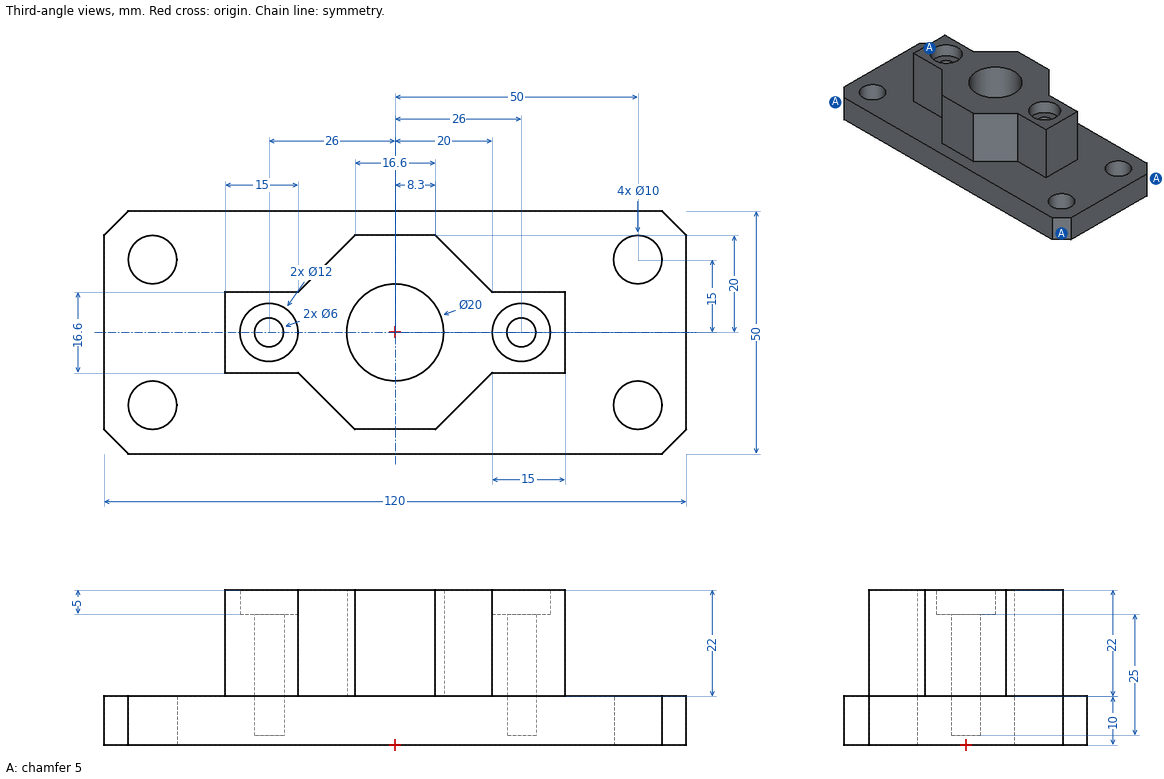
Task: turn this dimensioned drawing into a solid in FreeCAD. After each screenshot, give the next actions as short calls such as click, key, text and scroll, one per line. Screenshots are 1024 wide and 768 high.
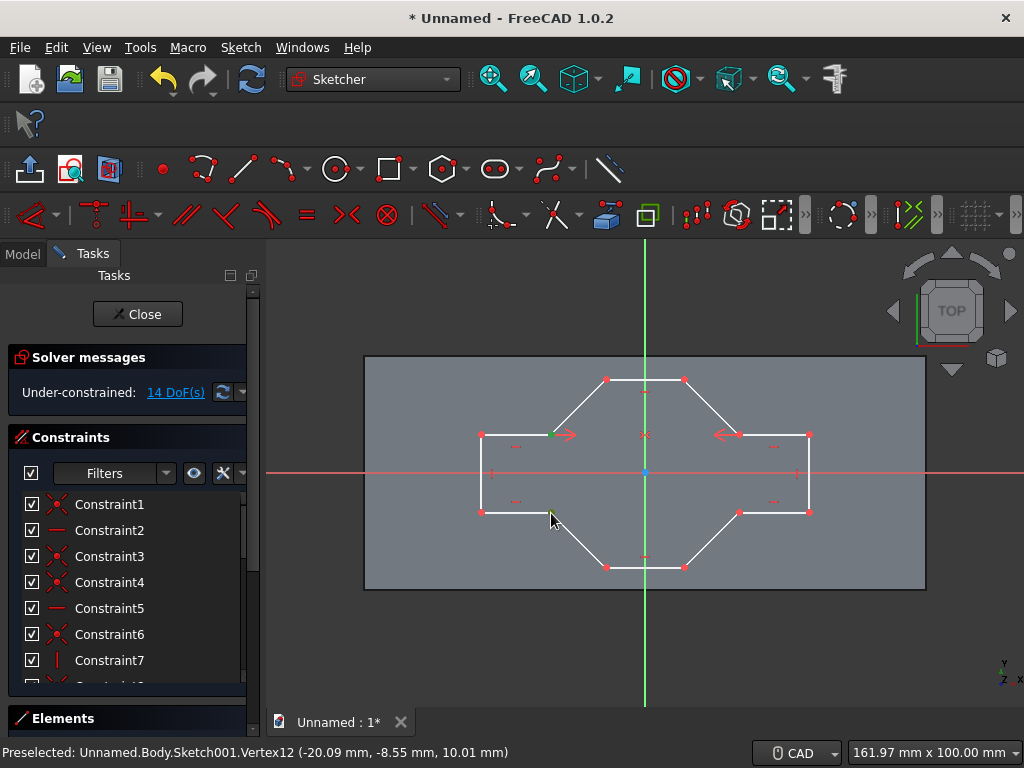
click(334, 473)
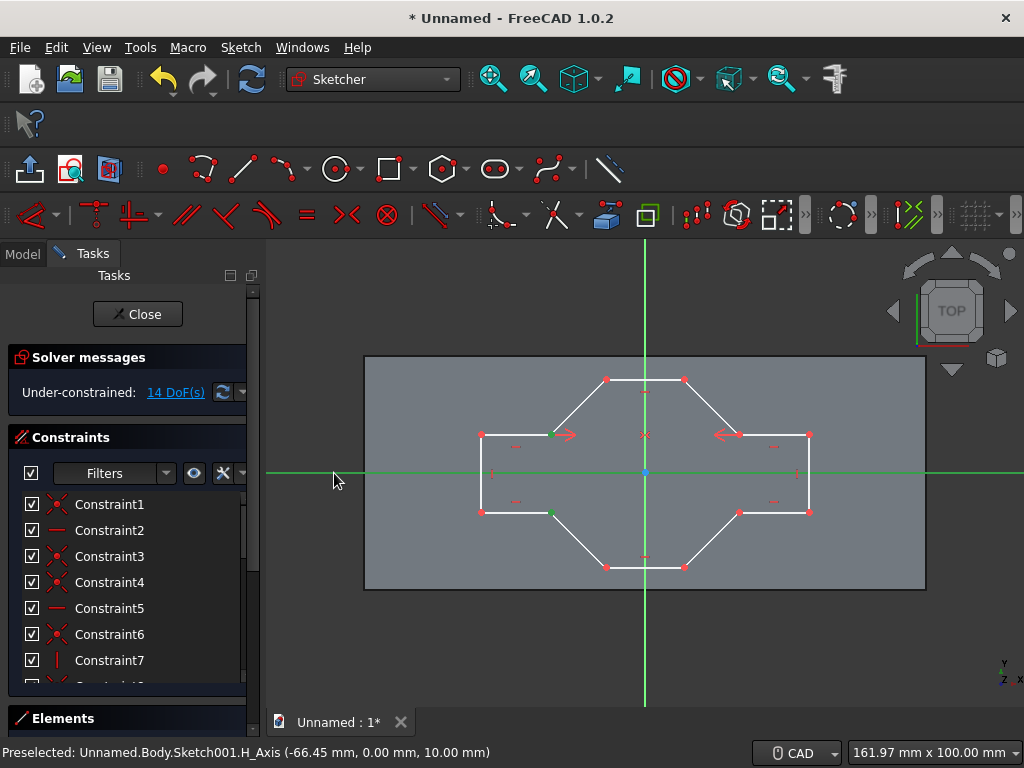
key(s)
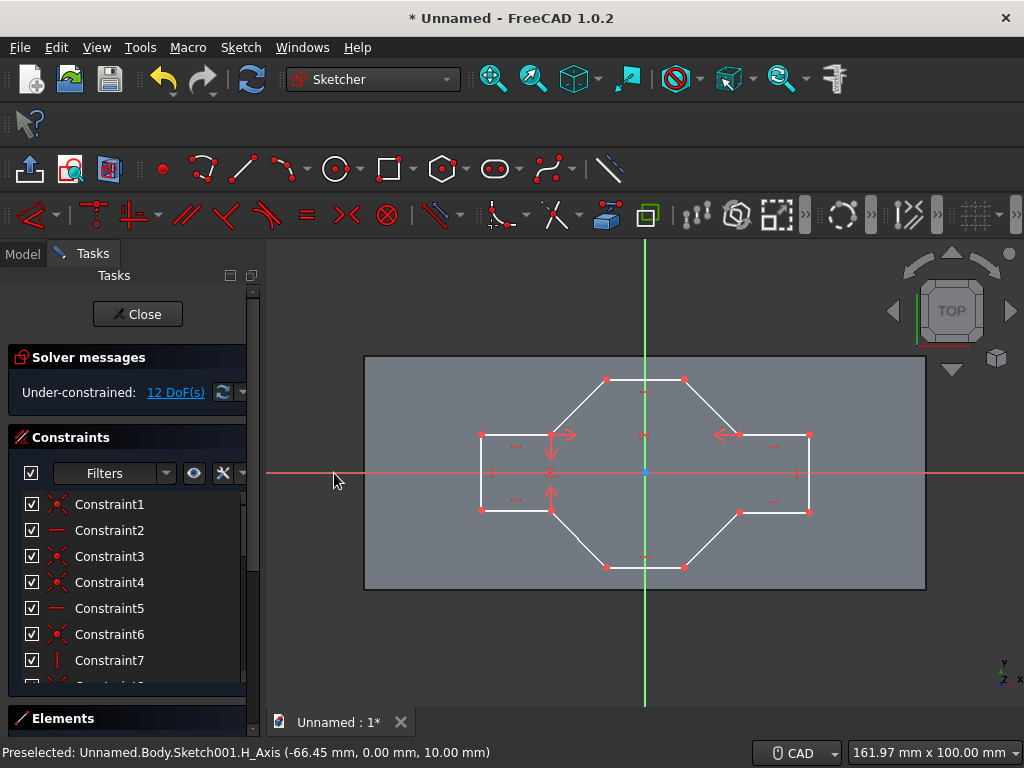
click(606, 380)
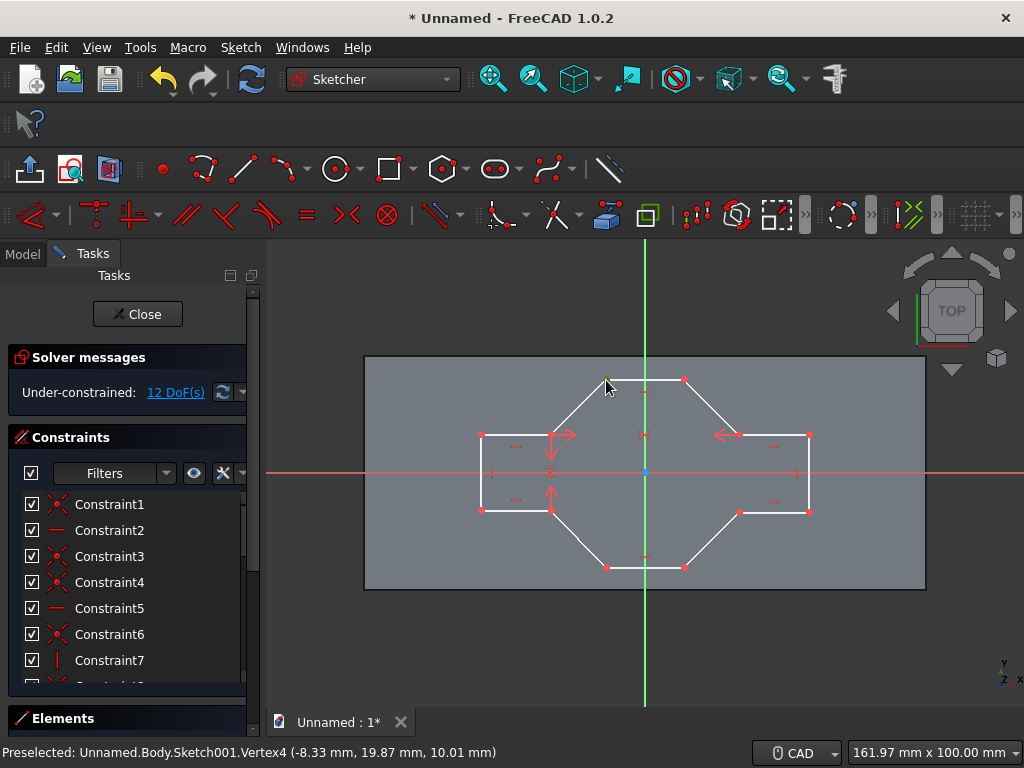
click(606, 568)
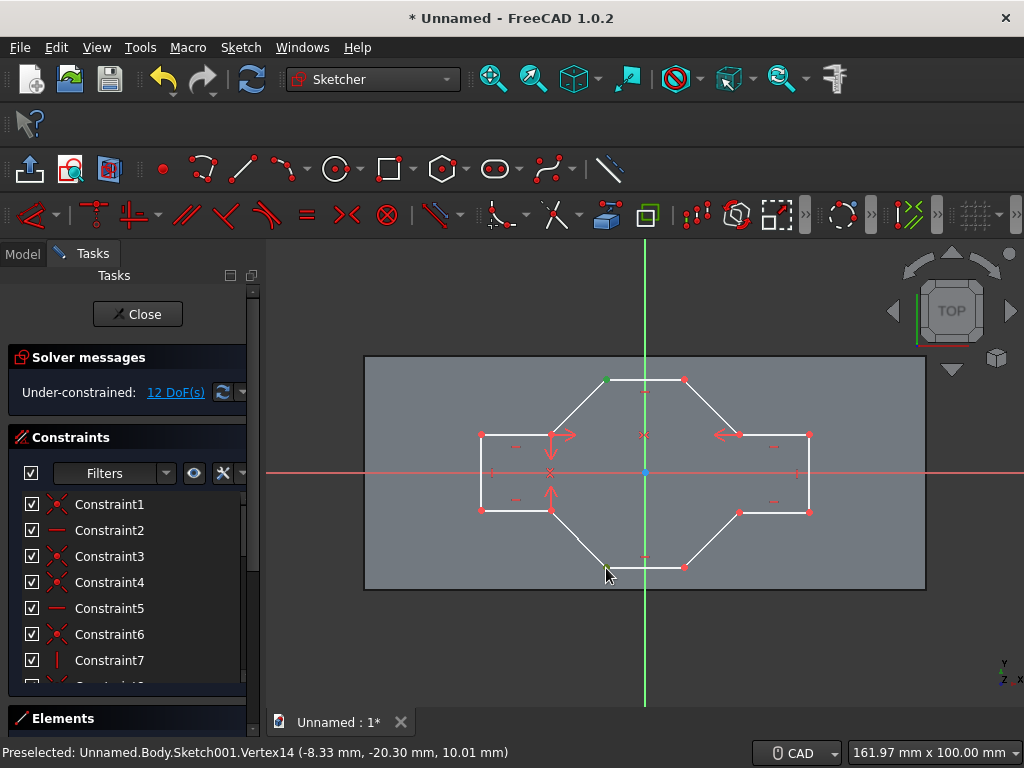
click(334, 473)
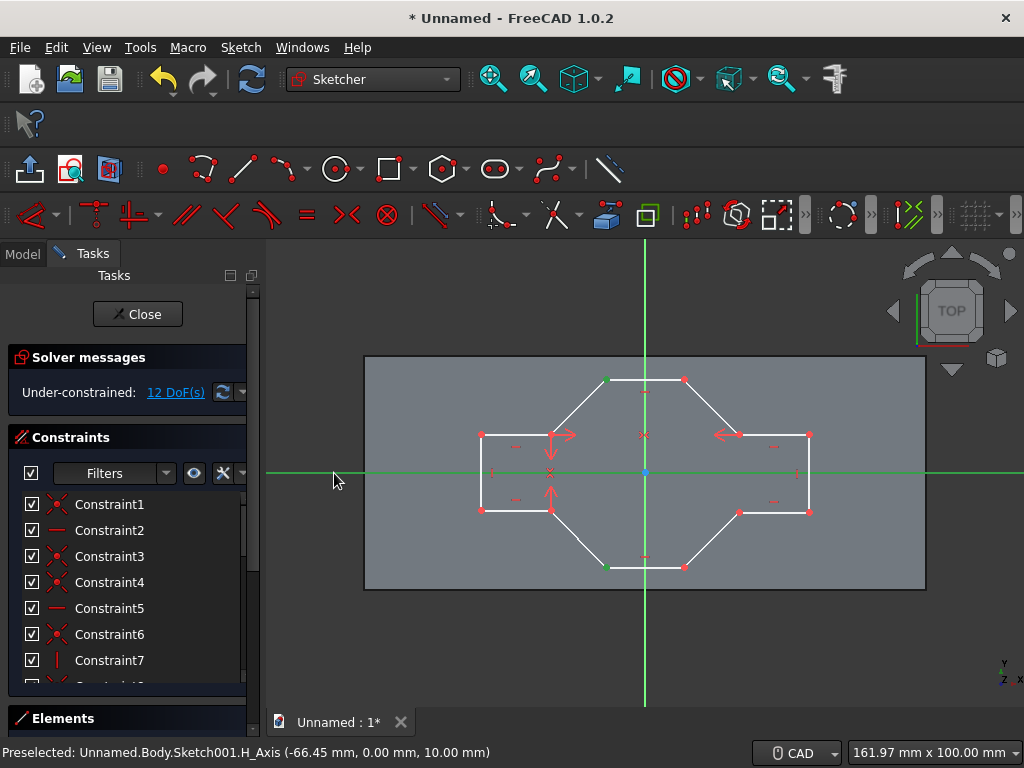
key(s)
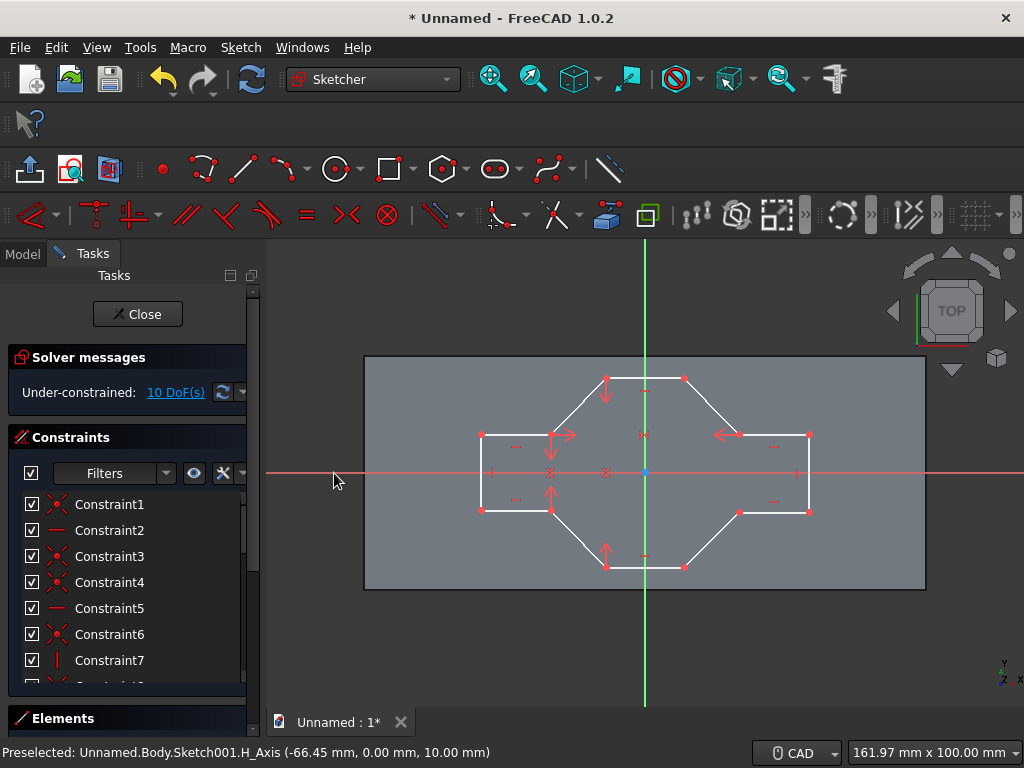
click(739, 435)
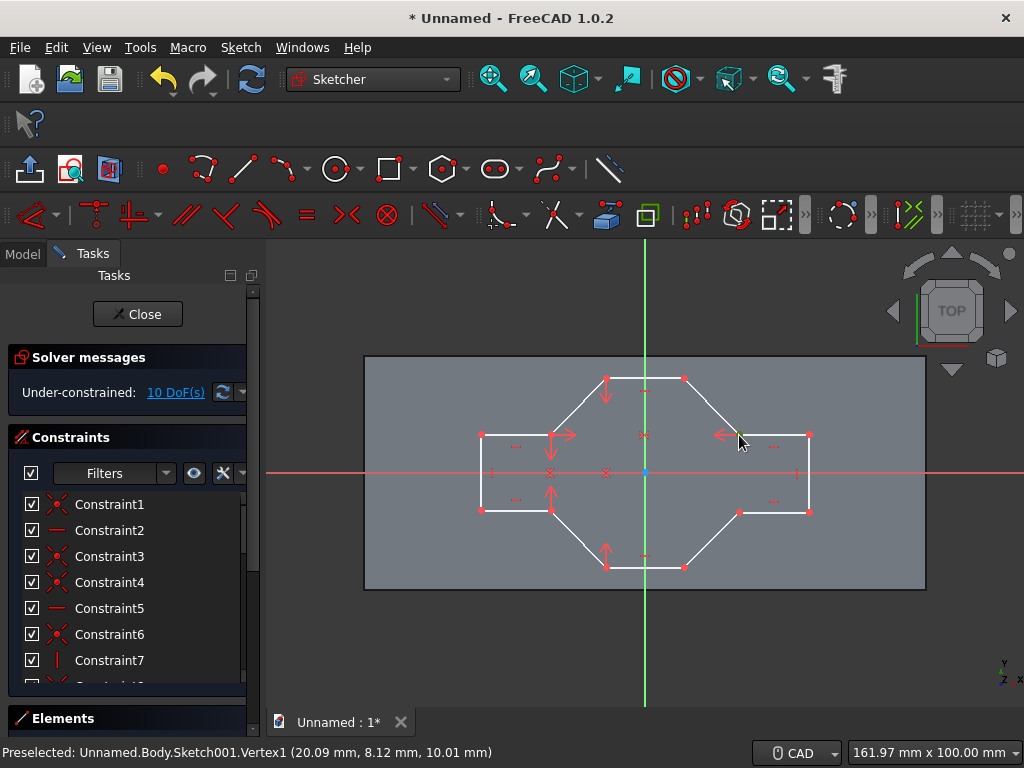
click(739, 513)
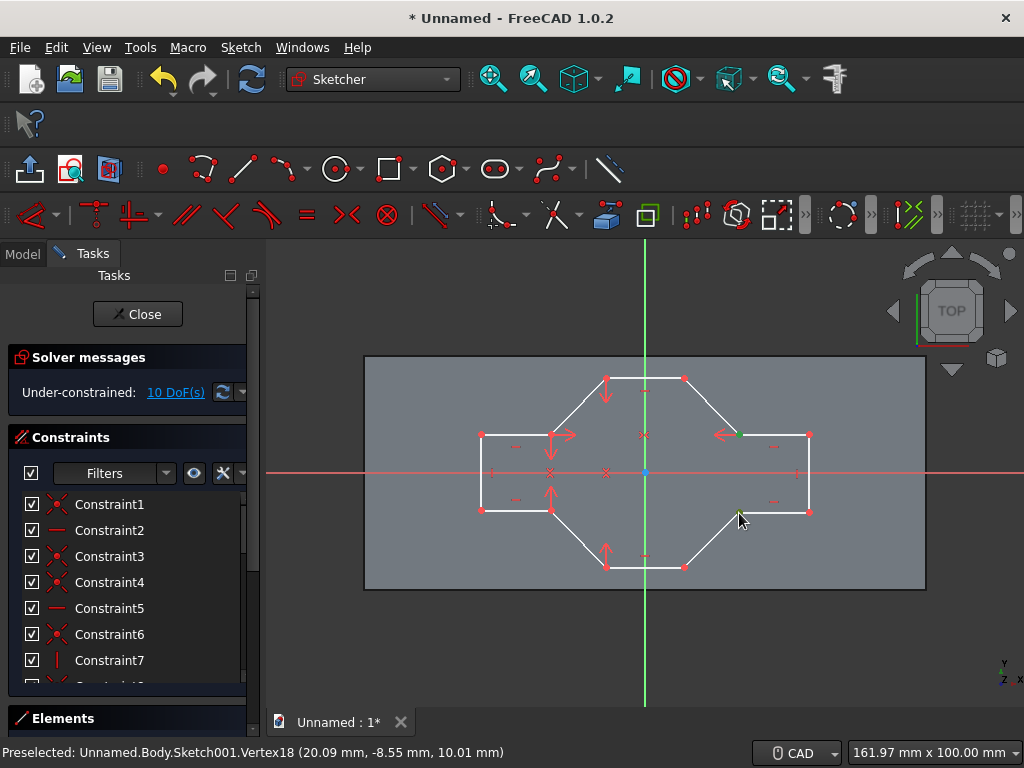
click(334, 473)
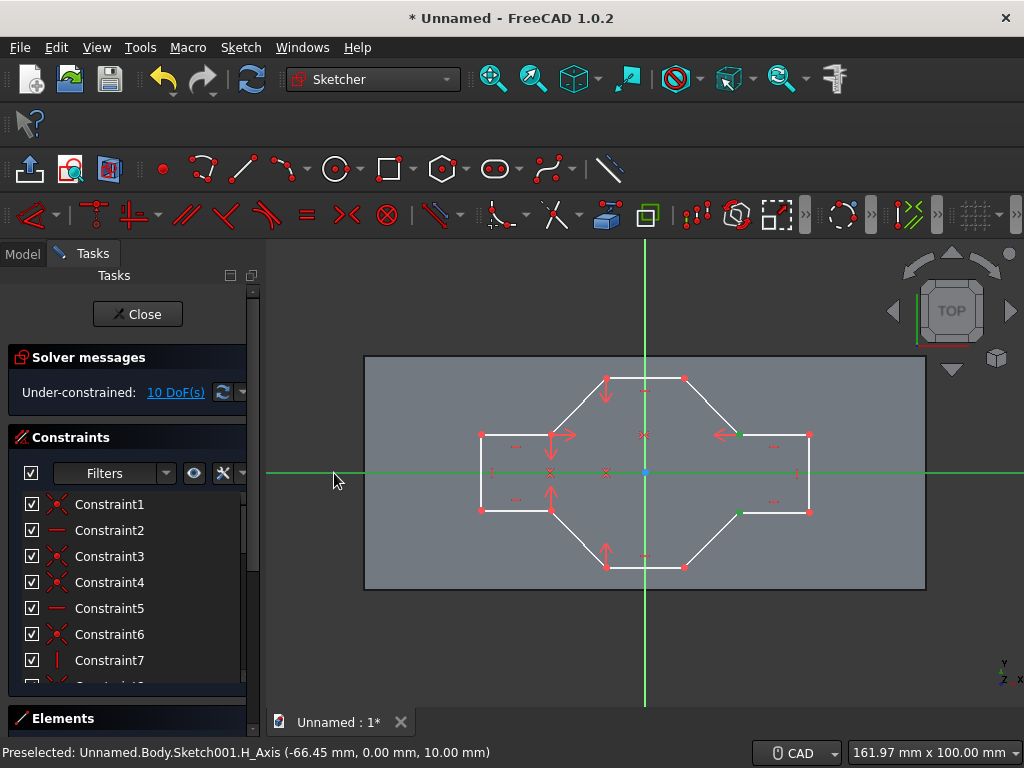
click(348, 216)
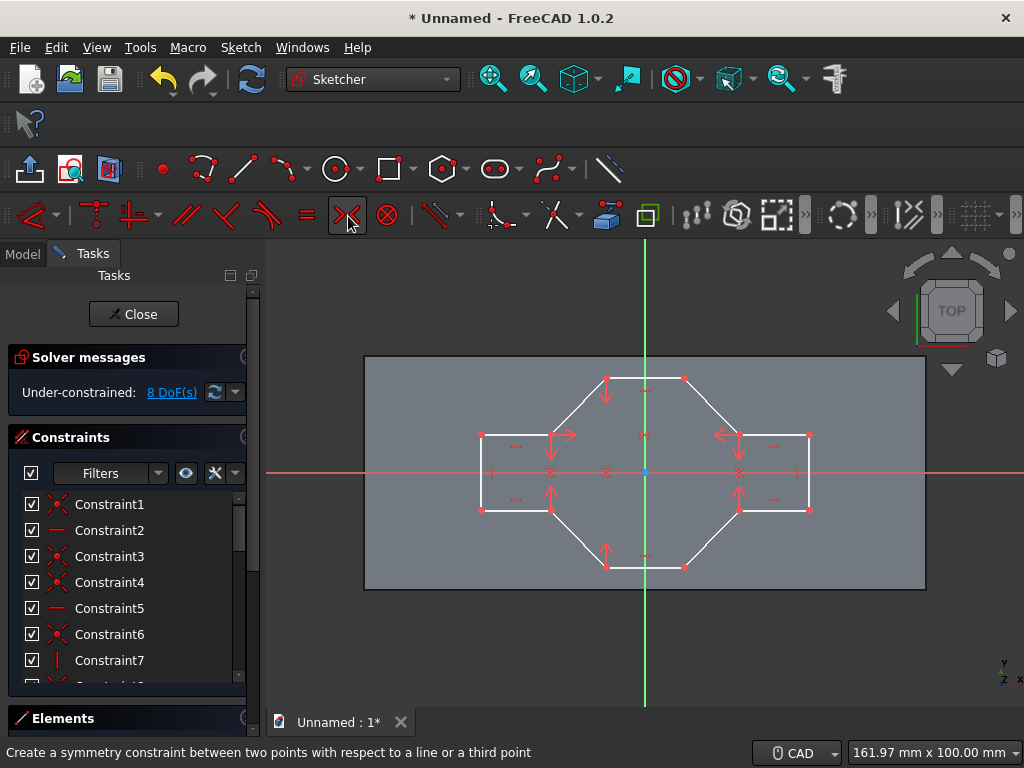
click(32, 216)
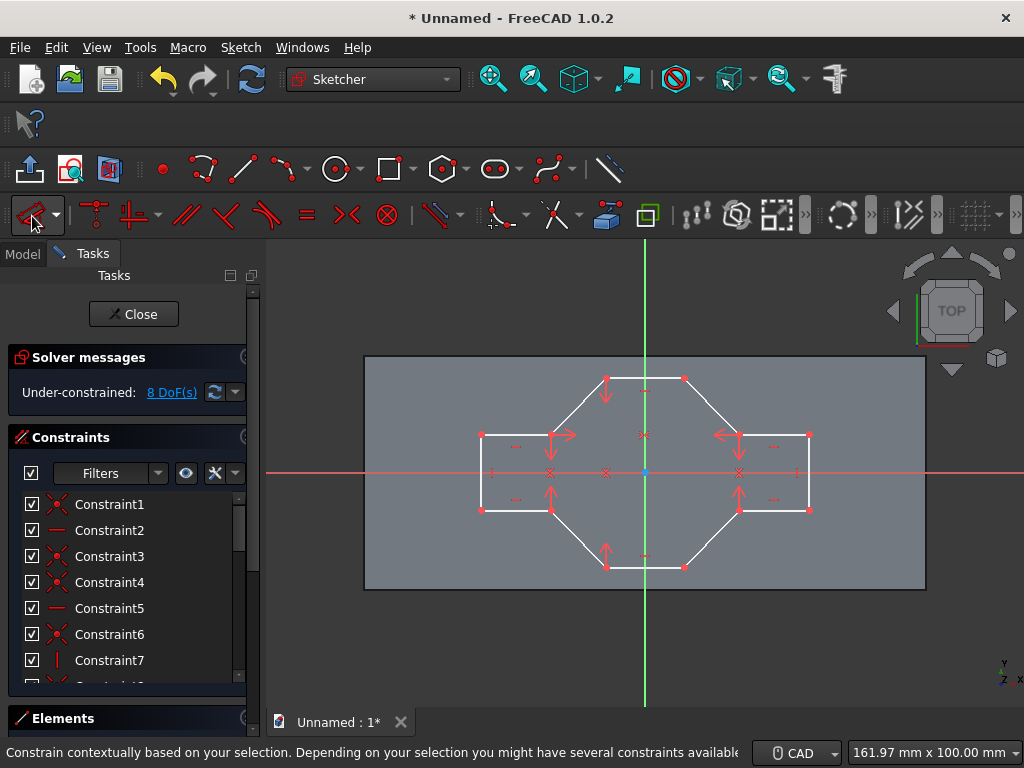
click(530, 435)
click(516, 401)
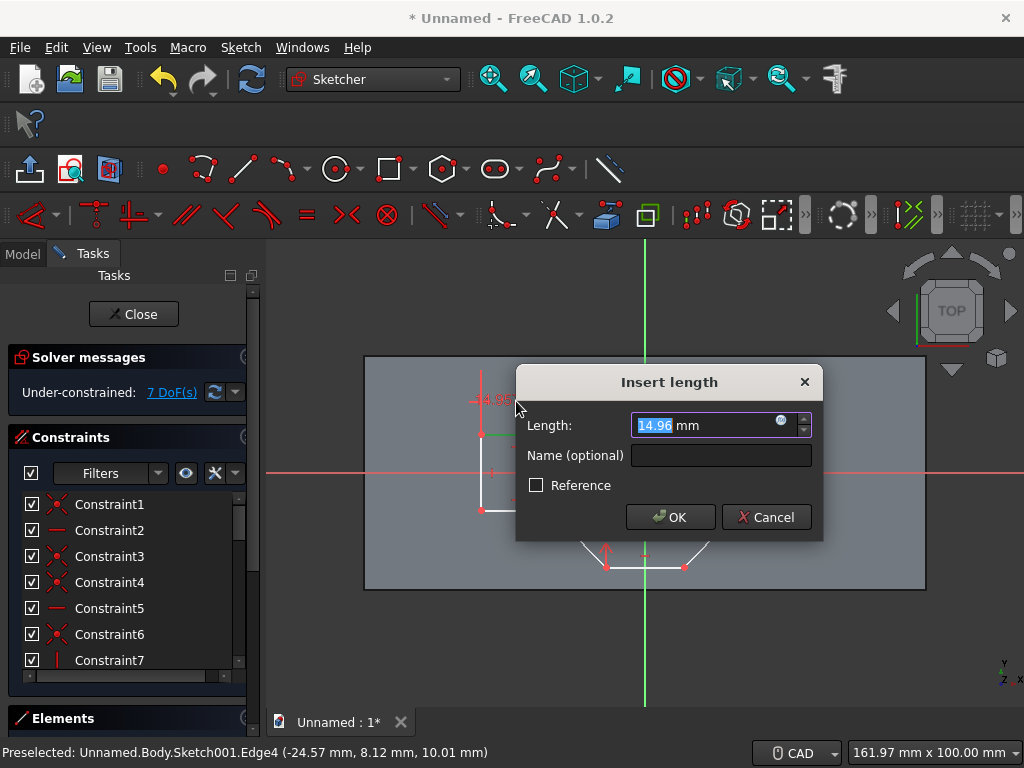
text(15)
key(Return)